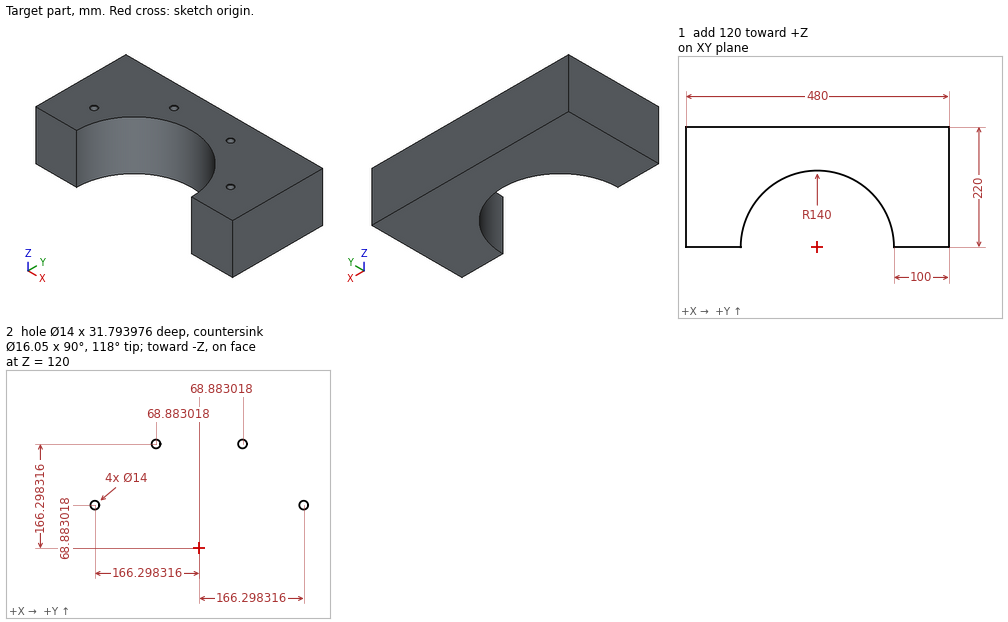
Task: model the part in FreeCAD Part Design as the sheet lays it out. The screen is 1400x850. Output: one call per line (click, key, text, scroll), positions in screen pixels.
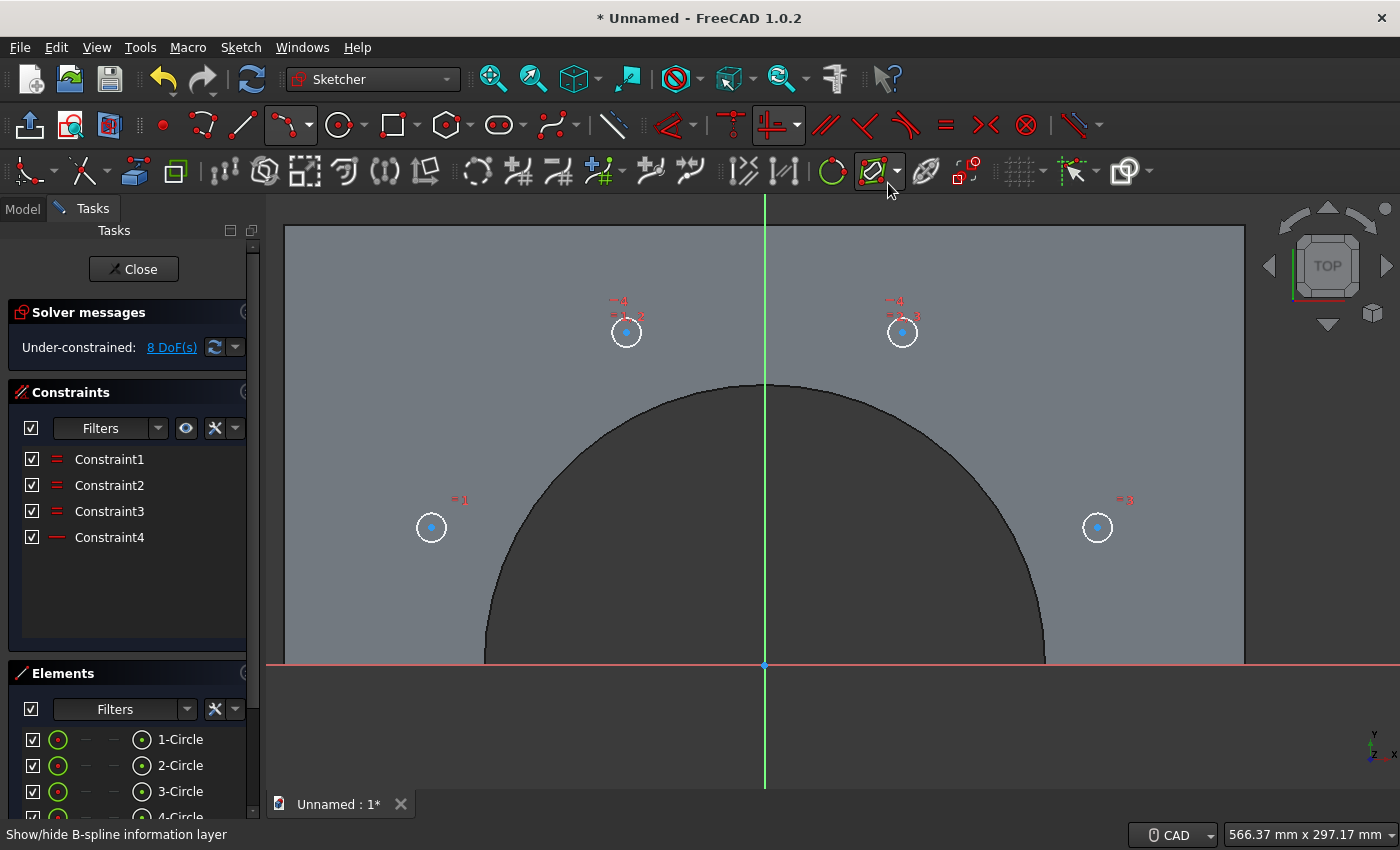
click(432, 528)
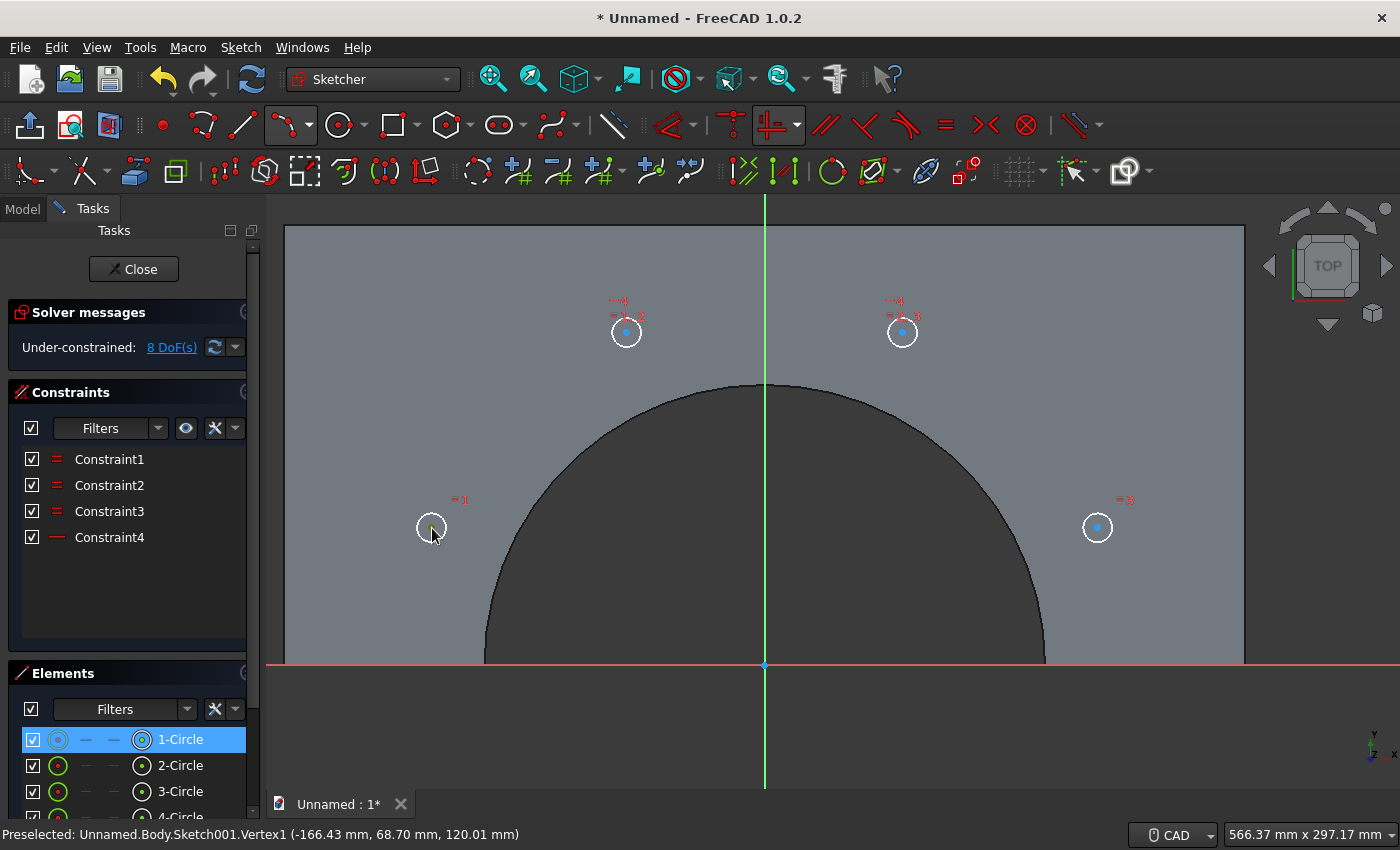
click(1098, 528)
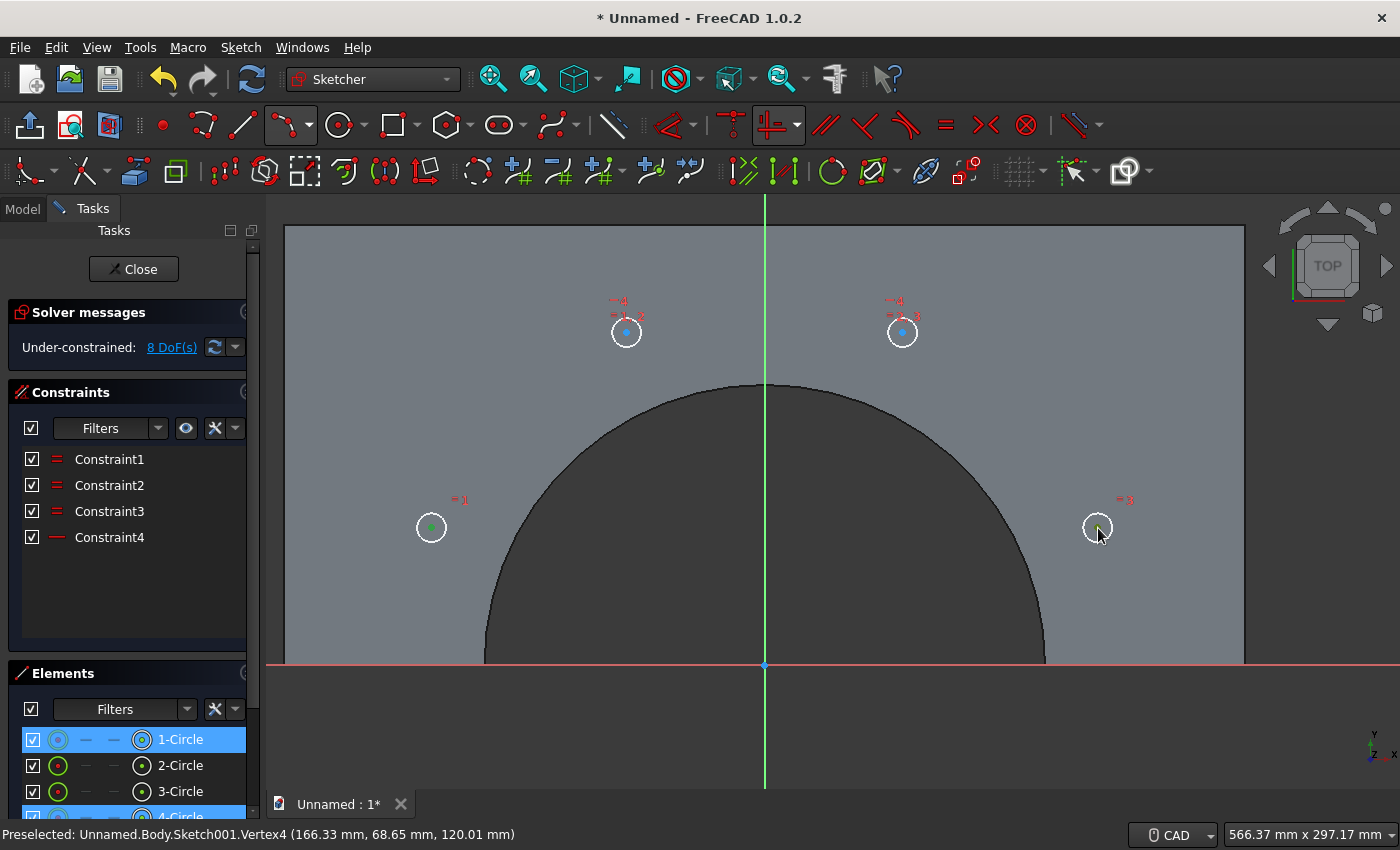
key(h)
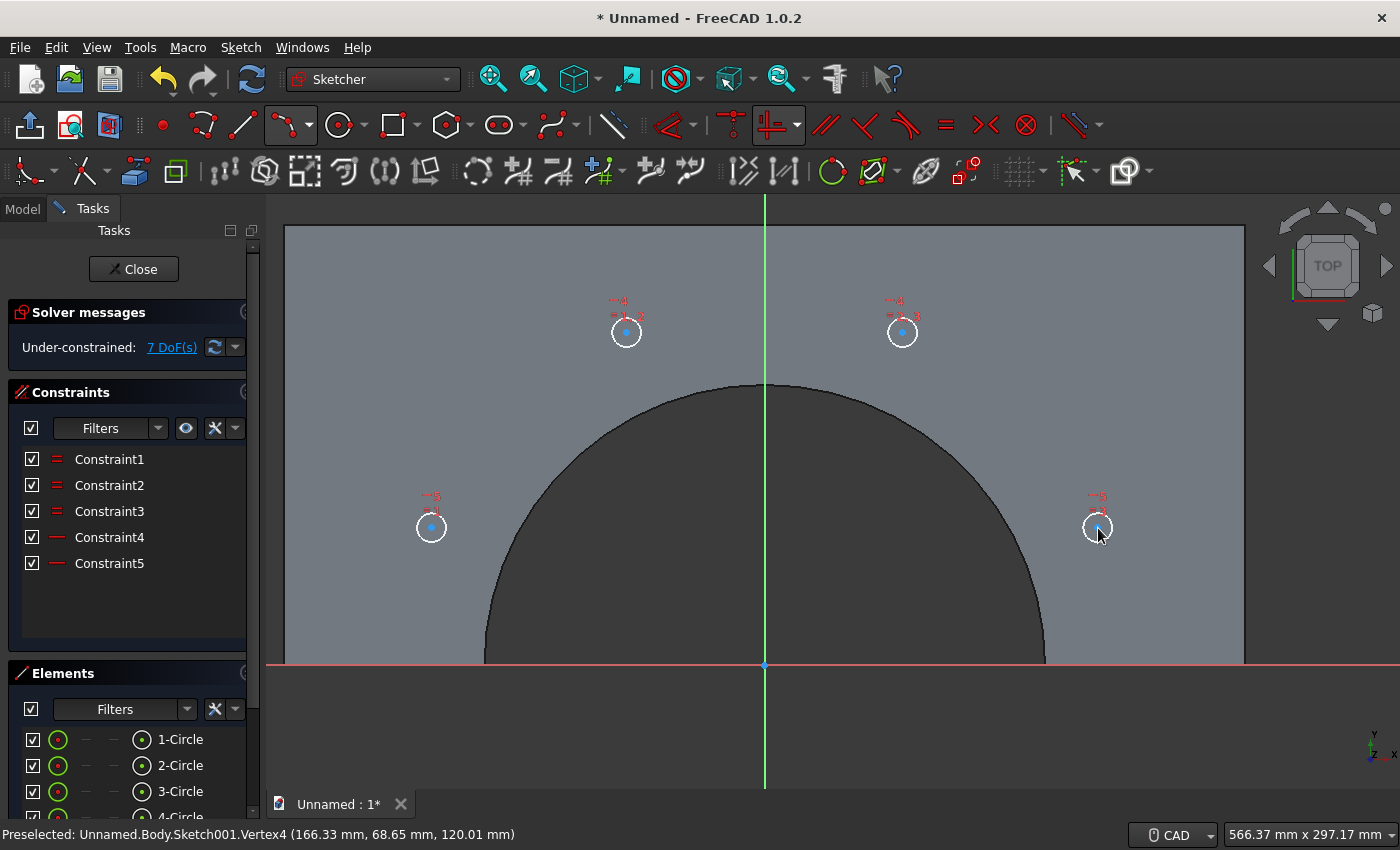
click(668, 126)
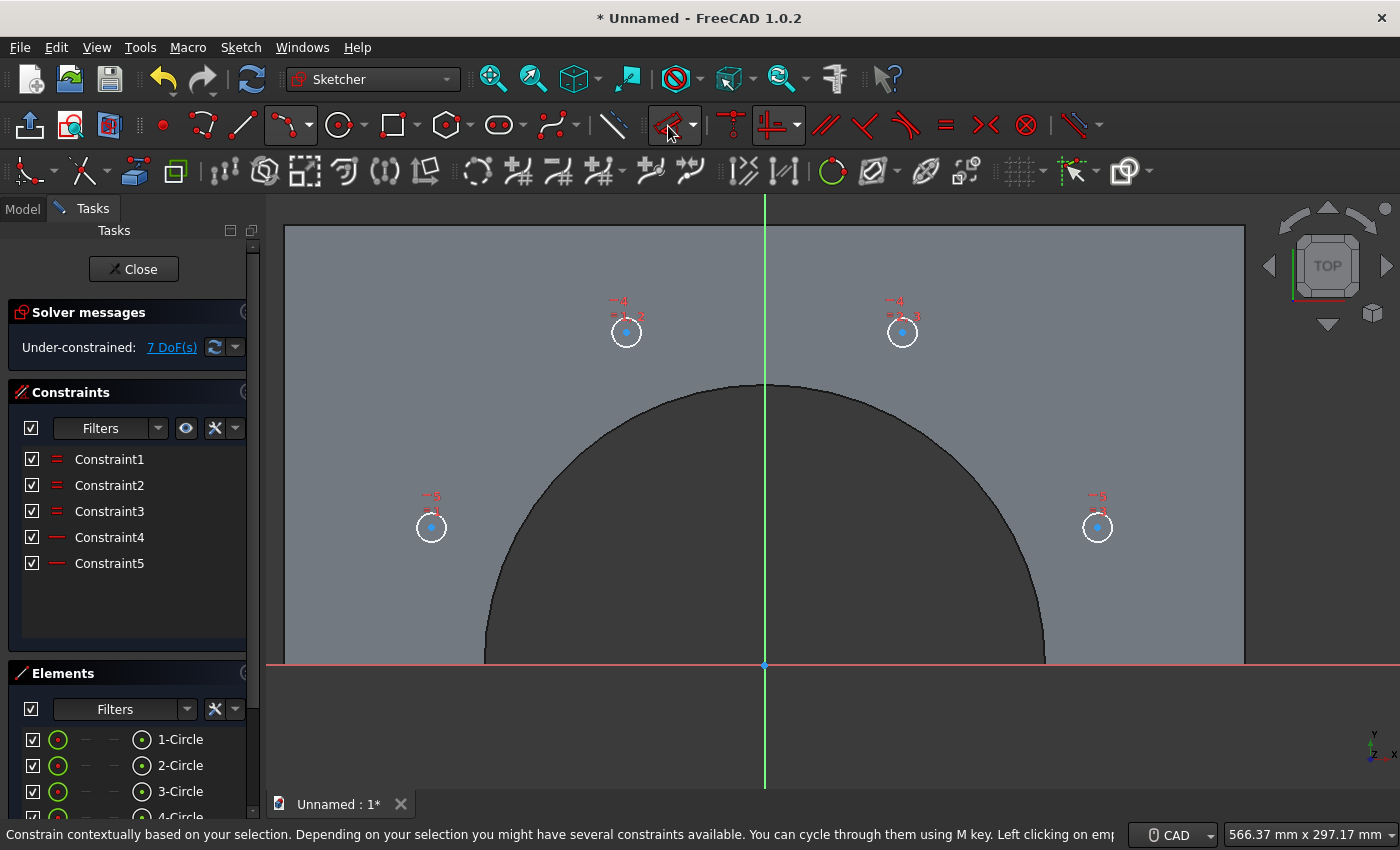
scroll(442, 518, up, 2)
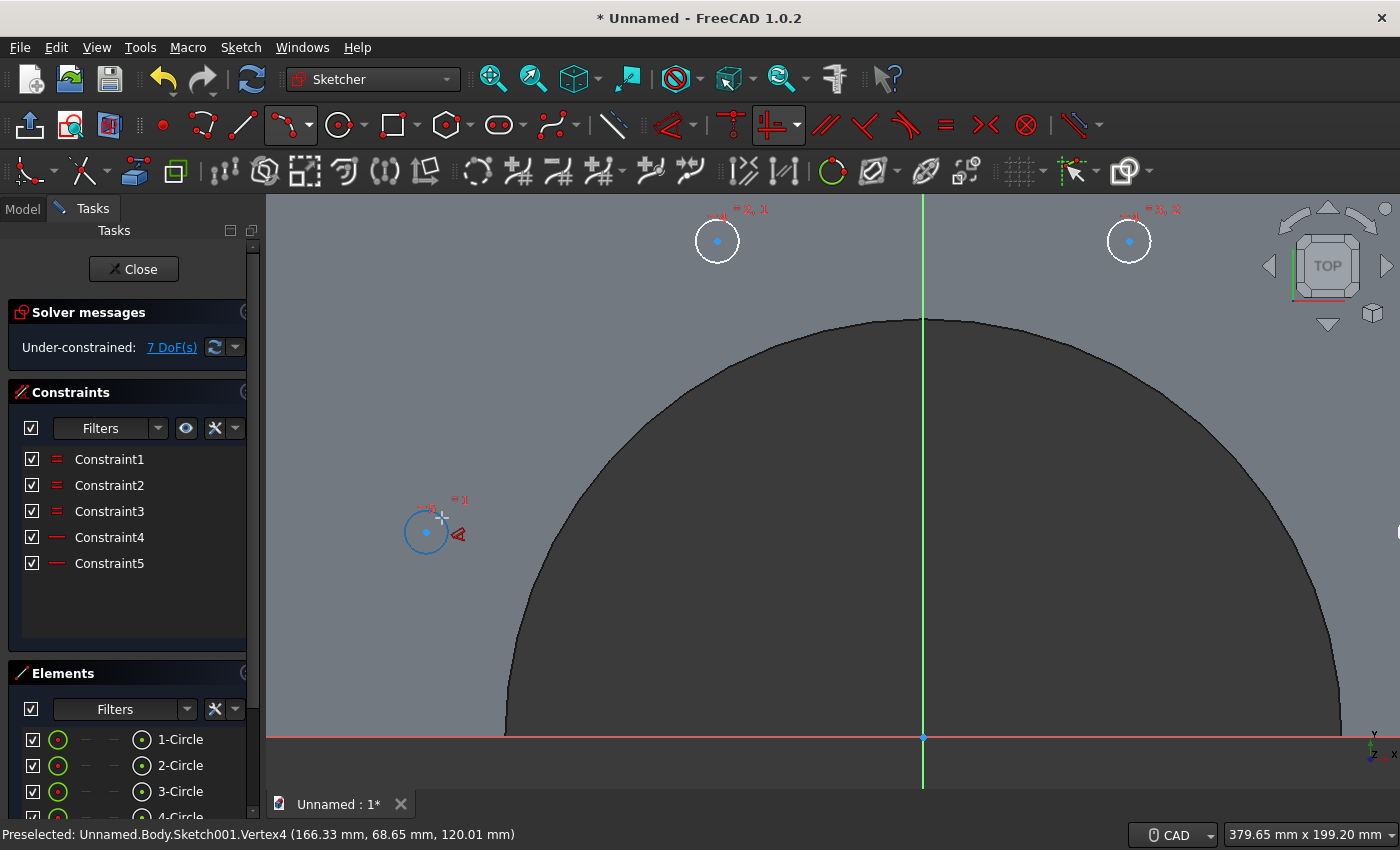
click(441, 517)
click(463, 494)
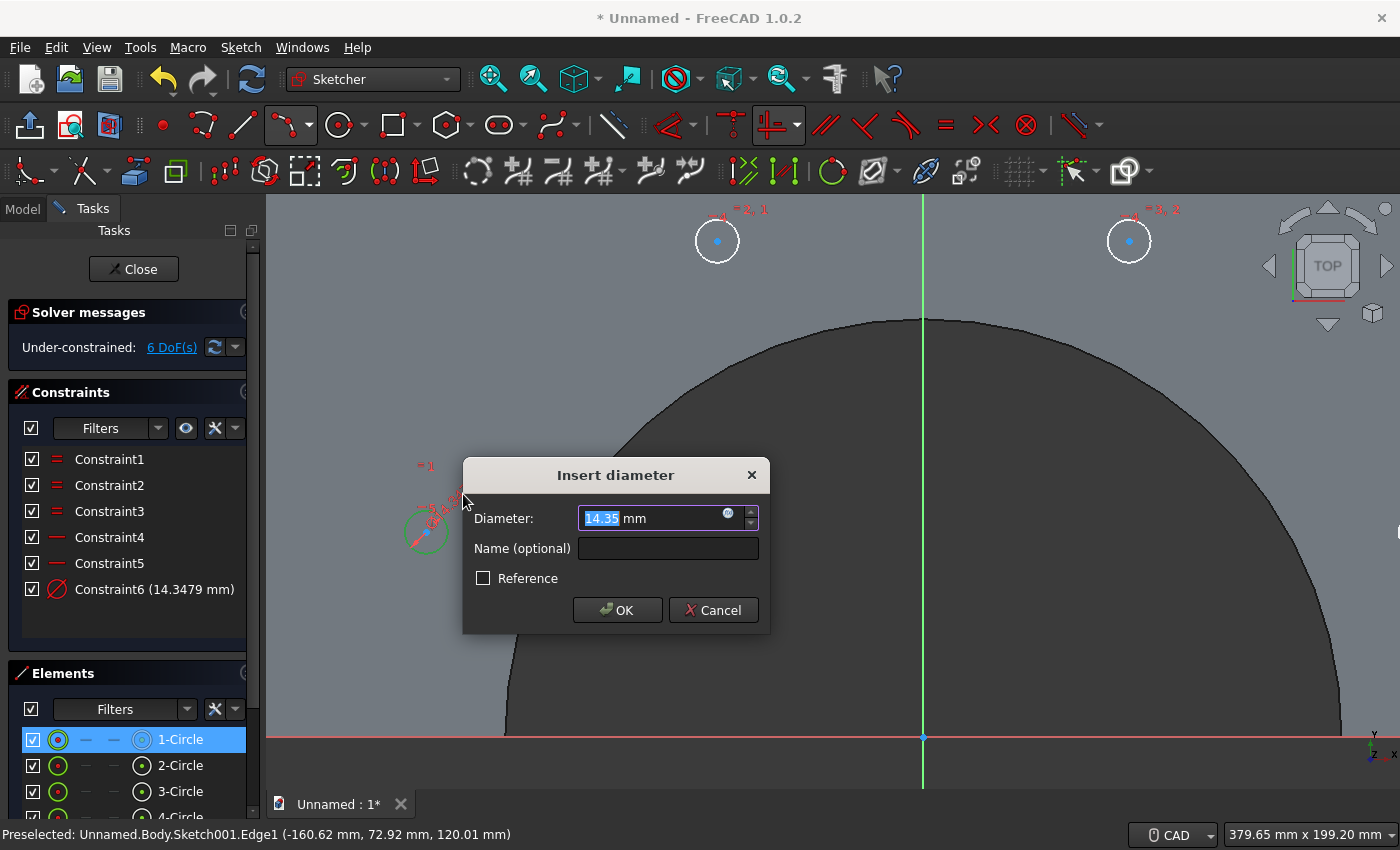
text(14)
key(Return)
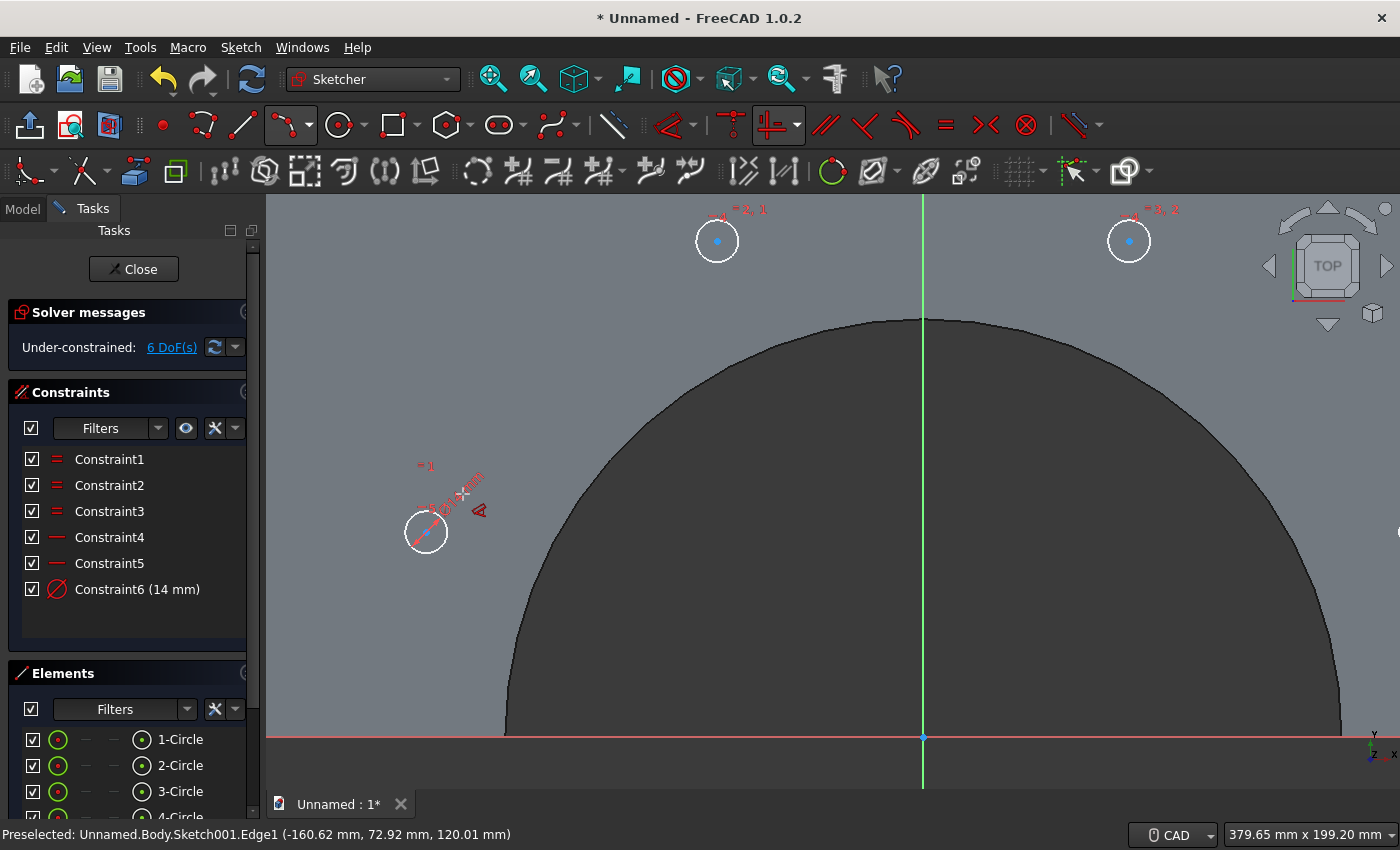
click(426, 532)
click(392, 635)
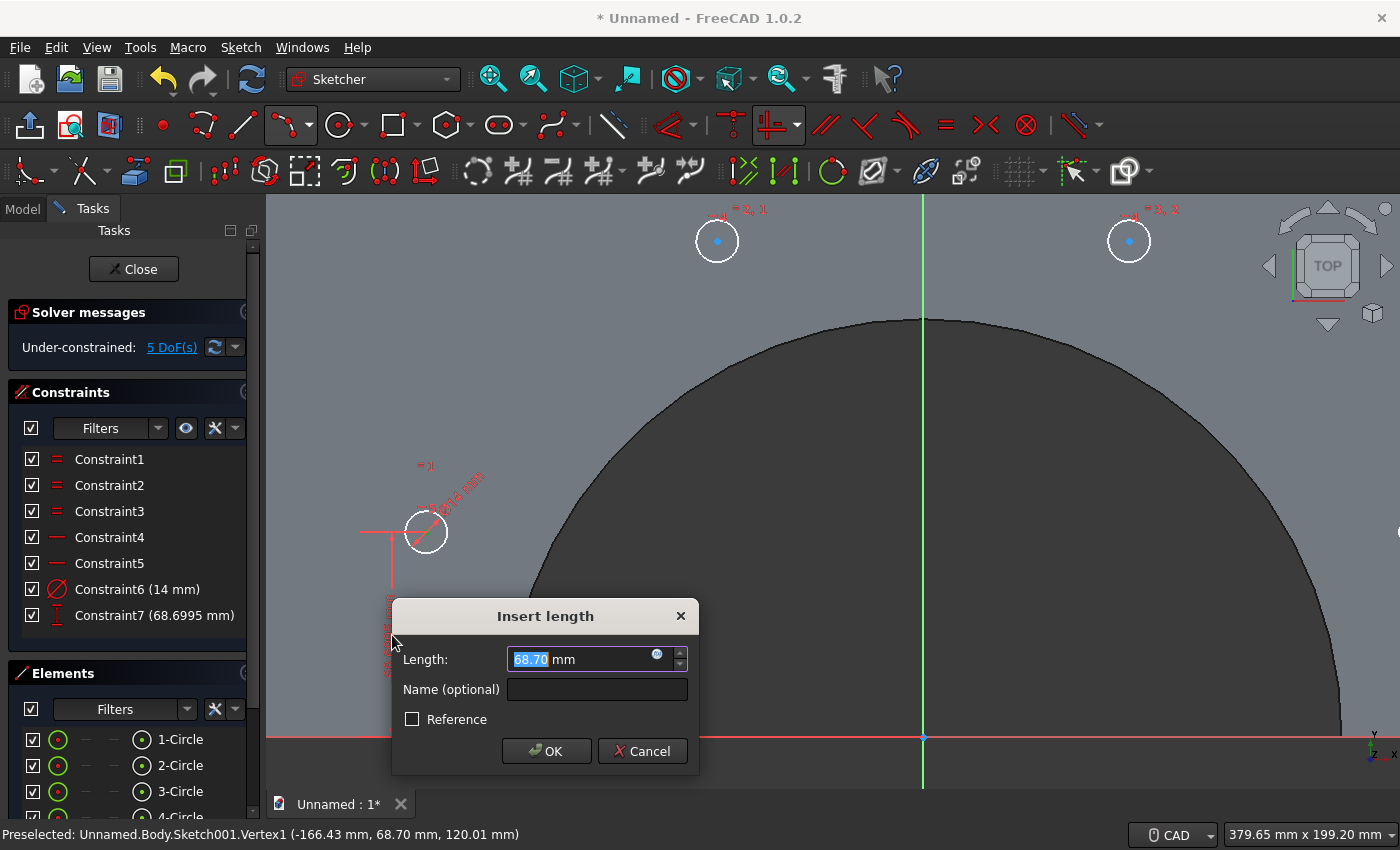
text(68.883018)
key(Return)